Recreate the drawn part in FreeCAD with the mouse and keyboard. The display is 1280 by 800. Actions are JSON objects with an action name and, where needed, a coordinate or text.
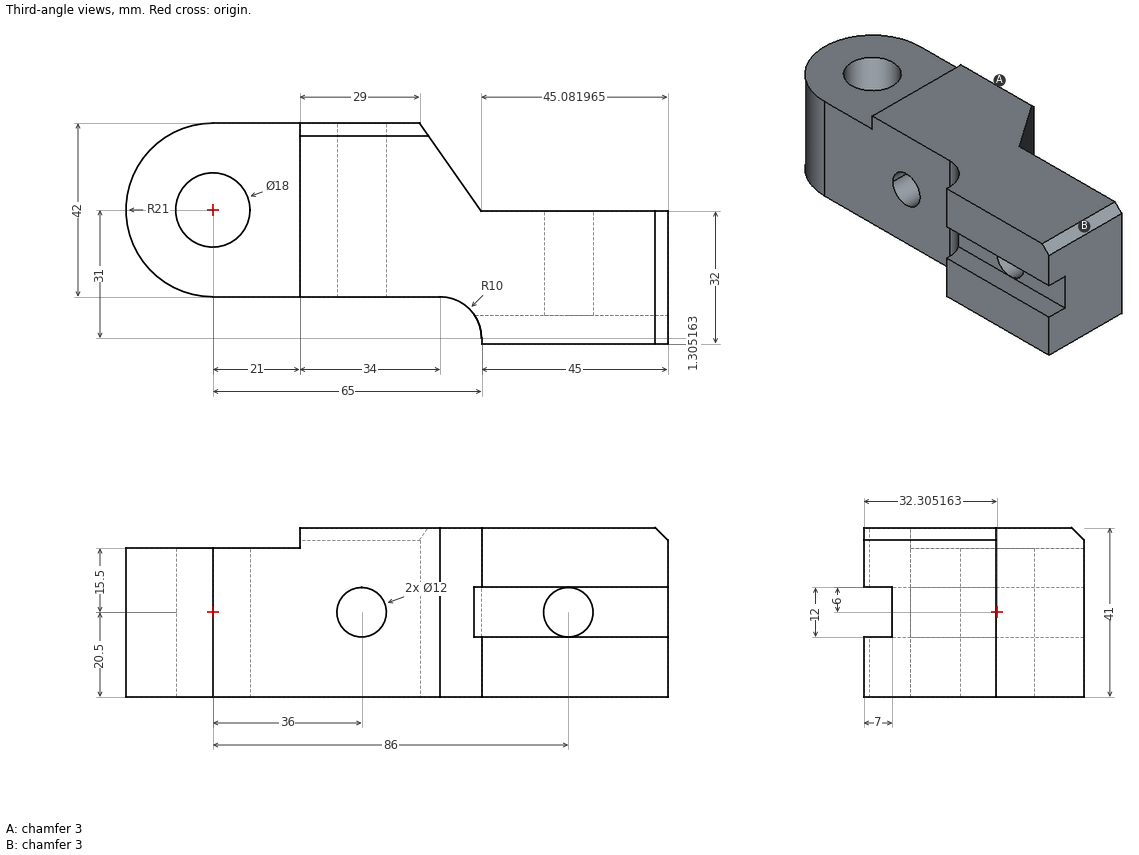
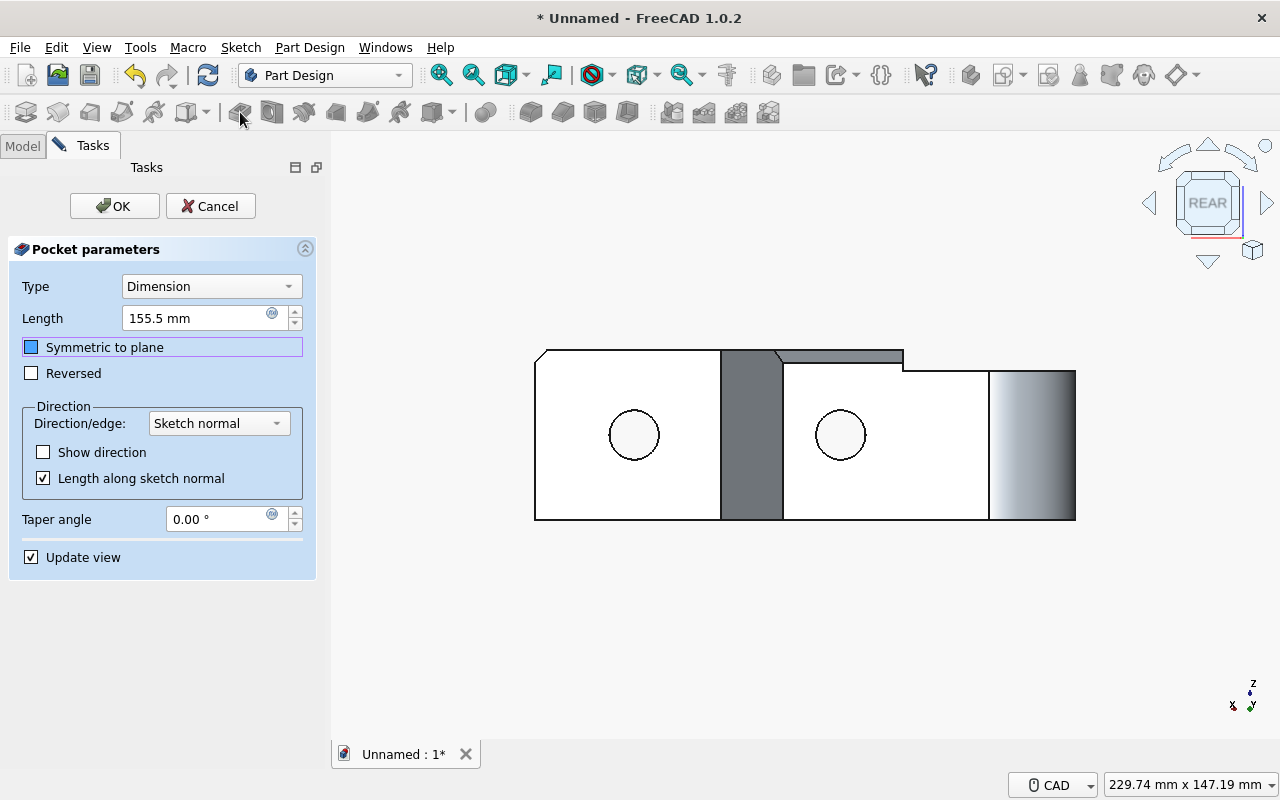
{"action": "left_click", "coordinate": [115, 206]}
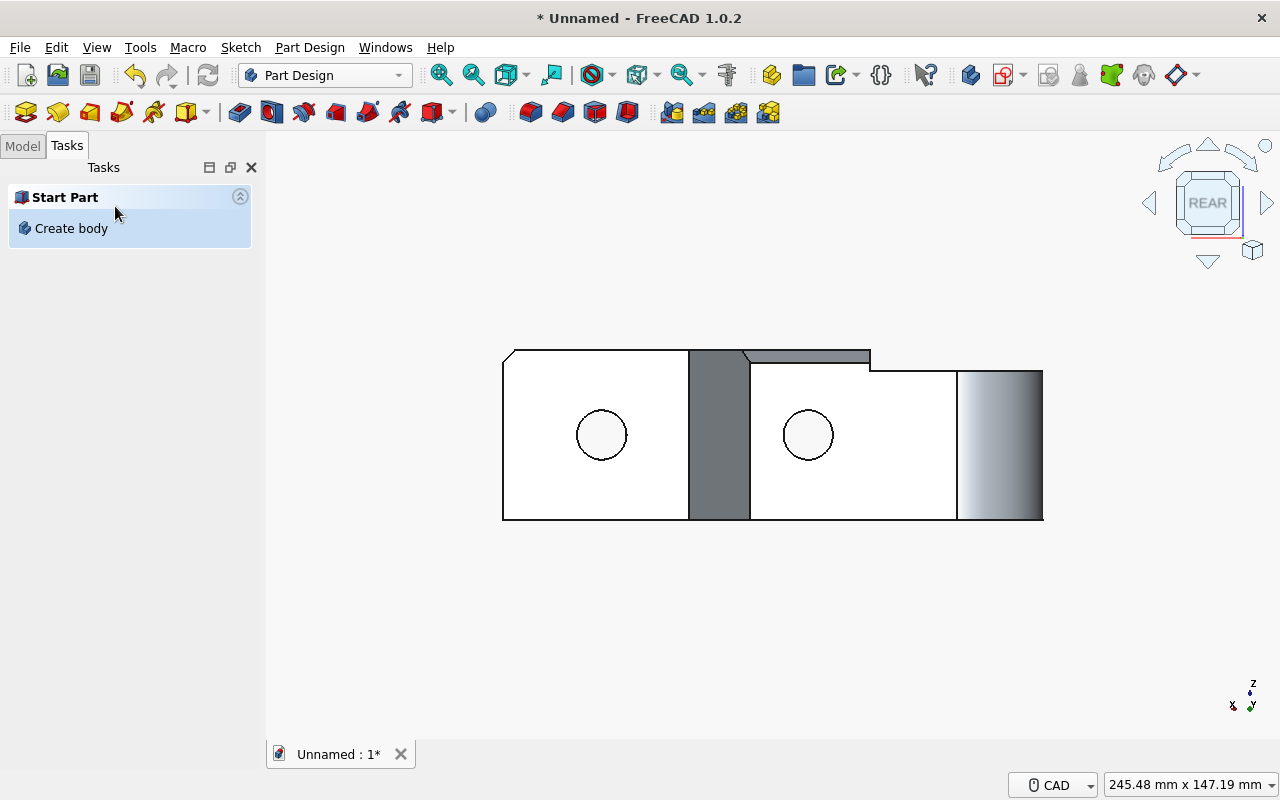
{"action": "key", "text": "0"}